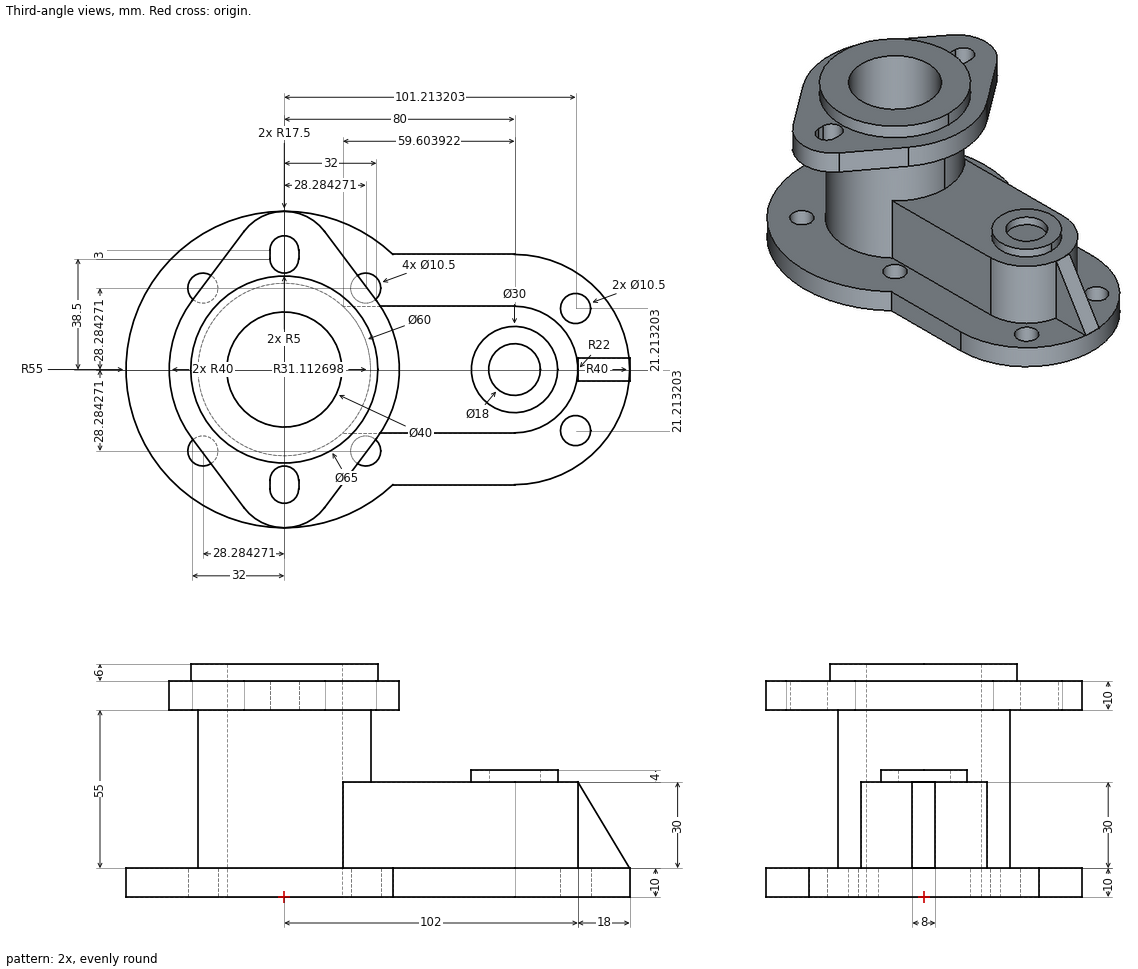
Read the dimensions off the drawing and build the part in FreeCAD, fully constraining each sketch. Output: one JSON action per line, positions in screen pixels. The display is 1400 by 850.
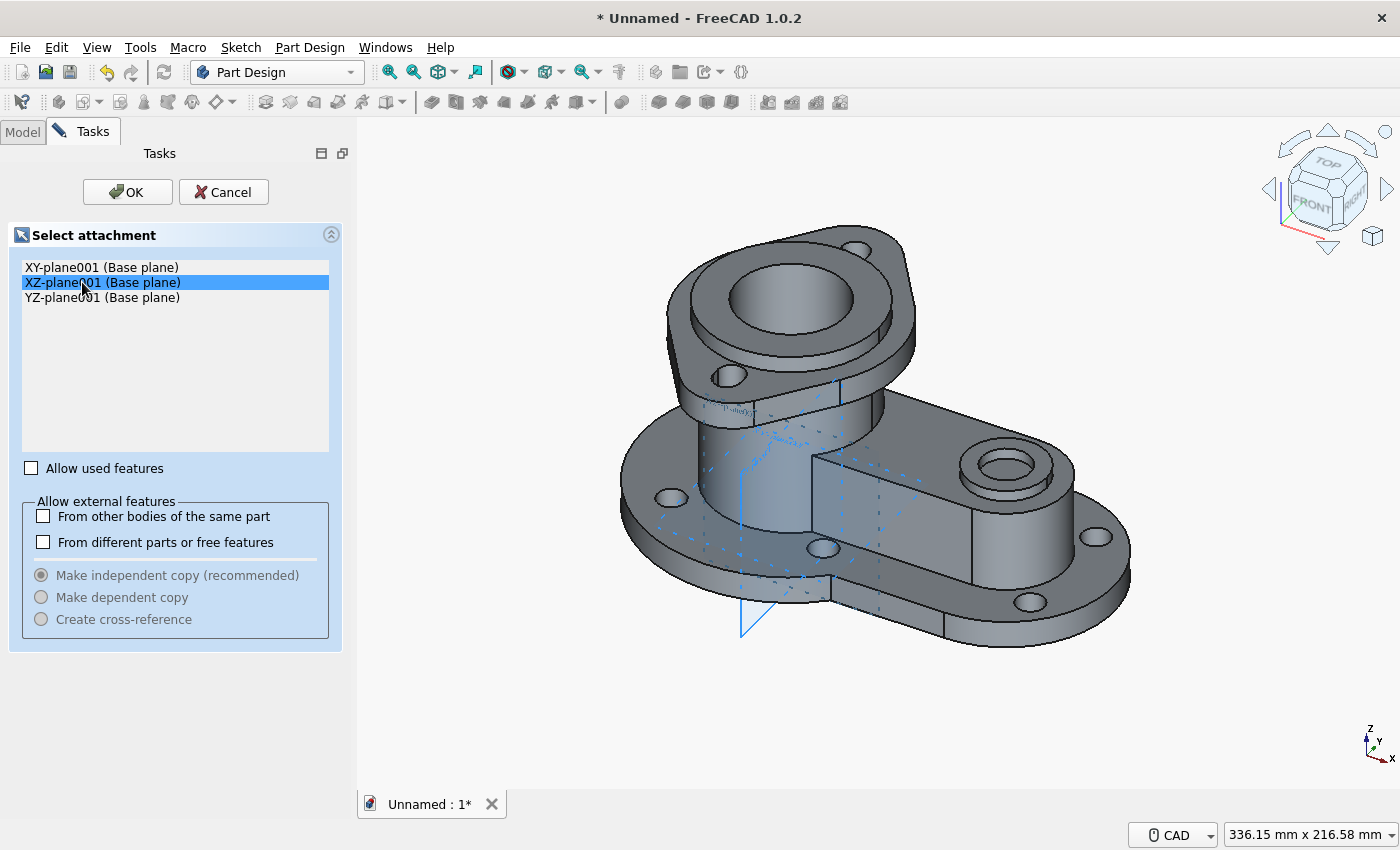
{"action": "left_click", "coordinate": [128, 192]}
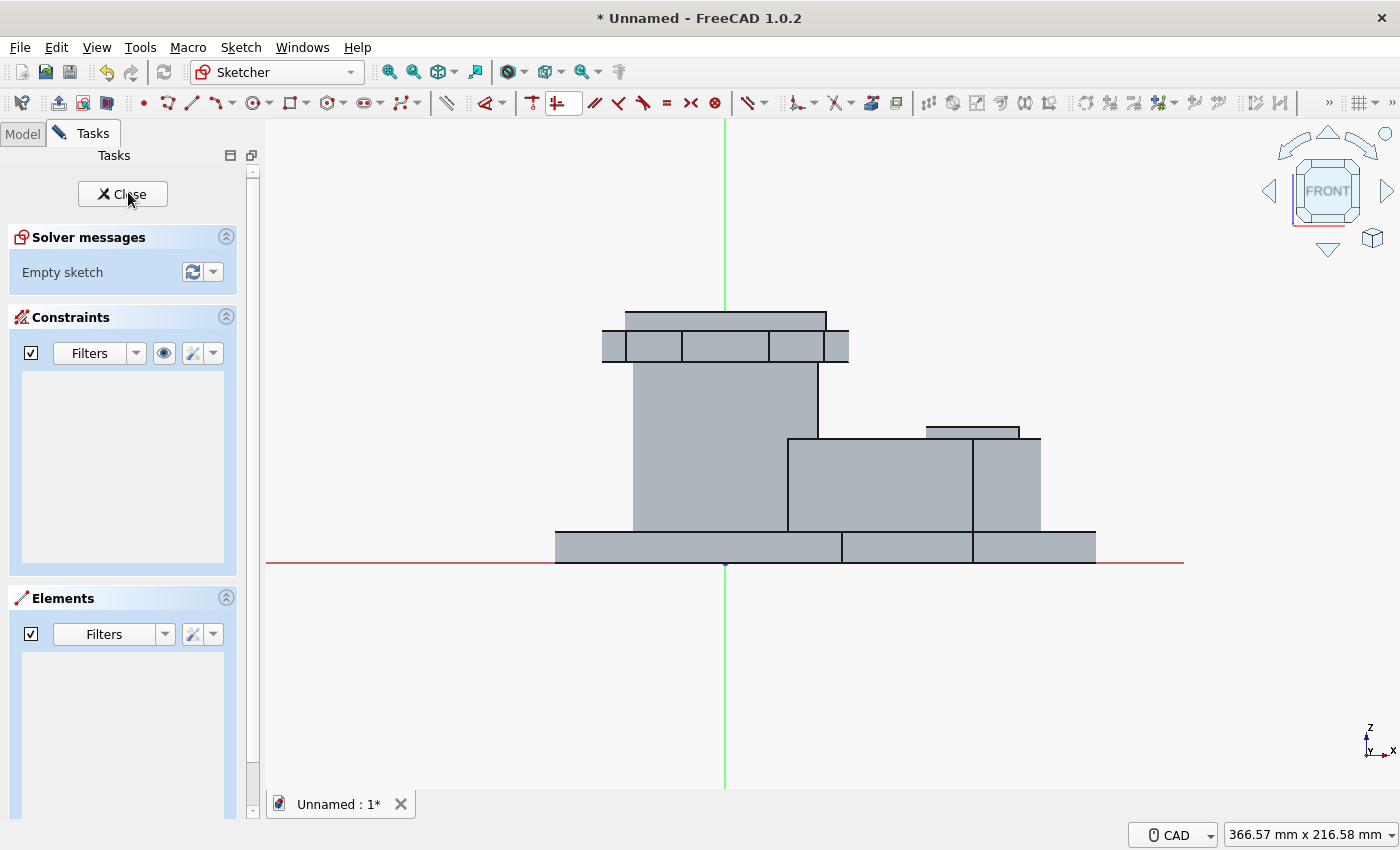
{"action": "scroll", "coordinate": [1146, 493], "scroll_direction": "up", "scroll_amount": 8}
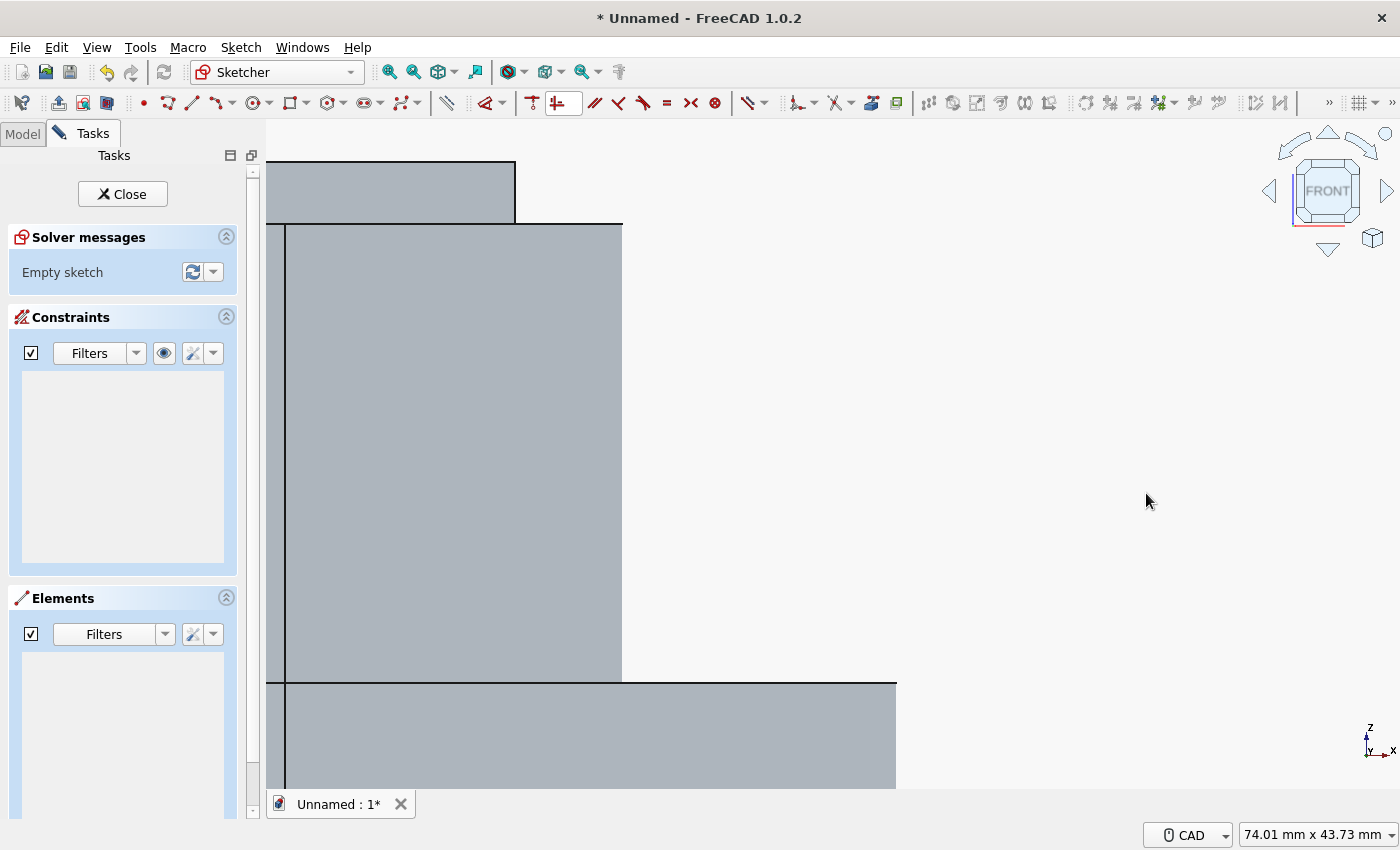
{"action": "left_click", "coordinate": [168, 104]}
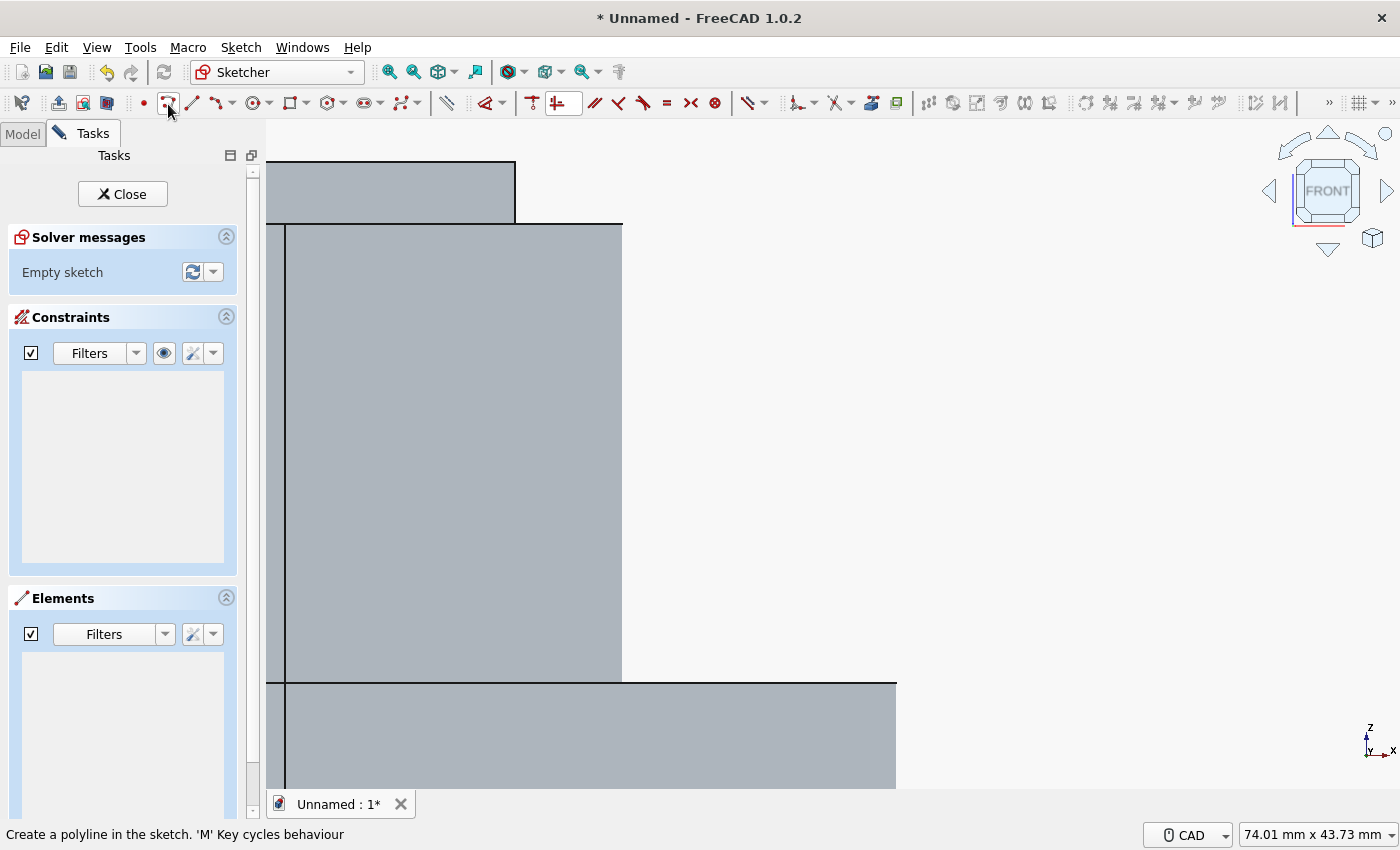
{"action": "left_click", "coordinate": [622, 683]}
{"action": "left_click", "coordinate": [622, 224]}
{"action": "left_click", "coordinate": [898, 683]}
{"action": "left_click", "coordinate": [622, 684]}
{"action": "key", "text": "Escape"}
{"action": "key", "text": "Escape"}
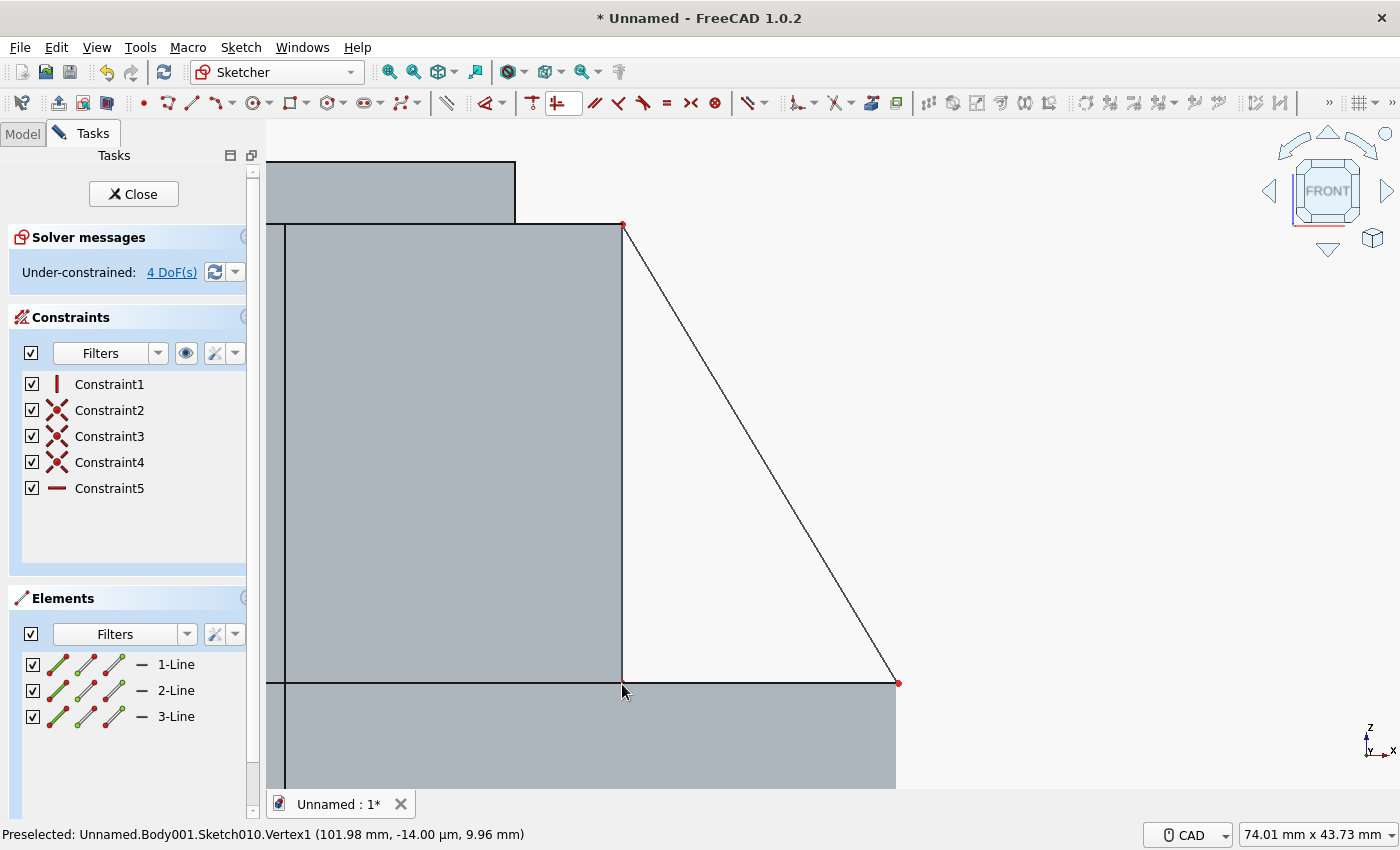
{"action": "key", "text": "d"}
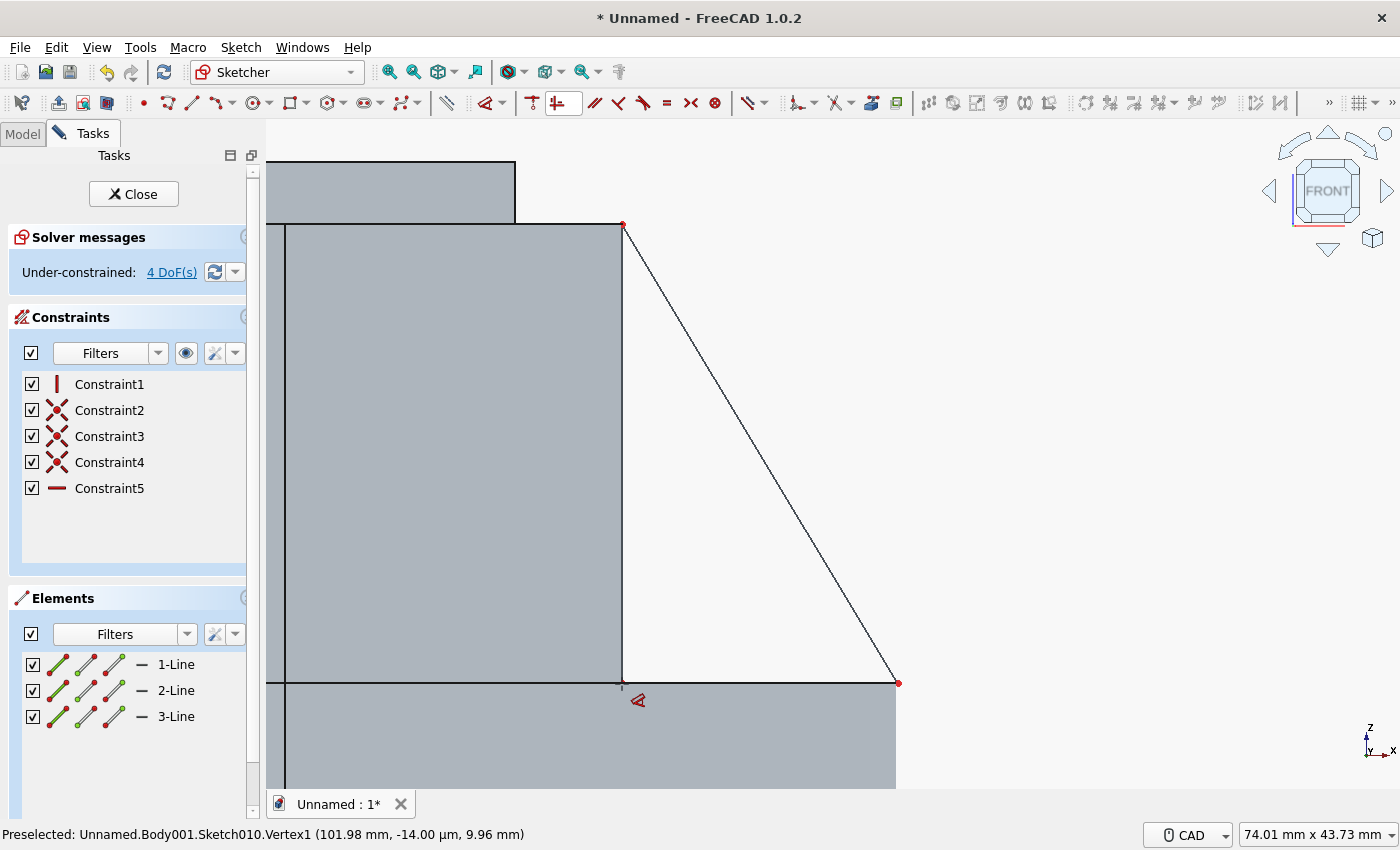
{"action": "left_click", "coordinate": [622, 546]}
{"action": "left_click", "coordinate": [588, 454]}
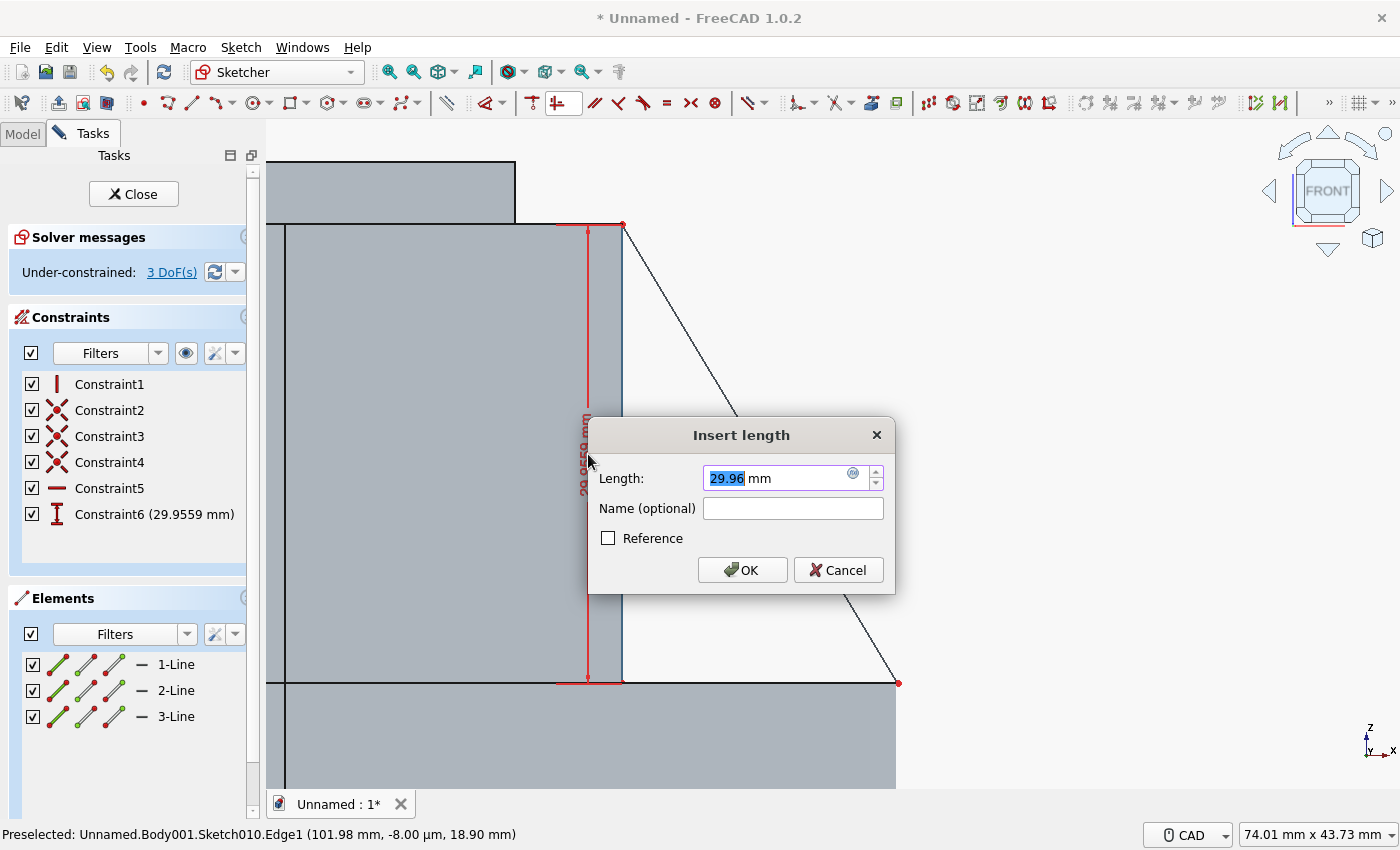
{"action": "type", "text": "30"}
{"action": "key", "text": "Return"}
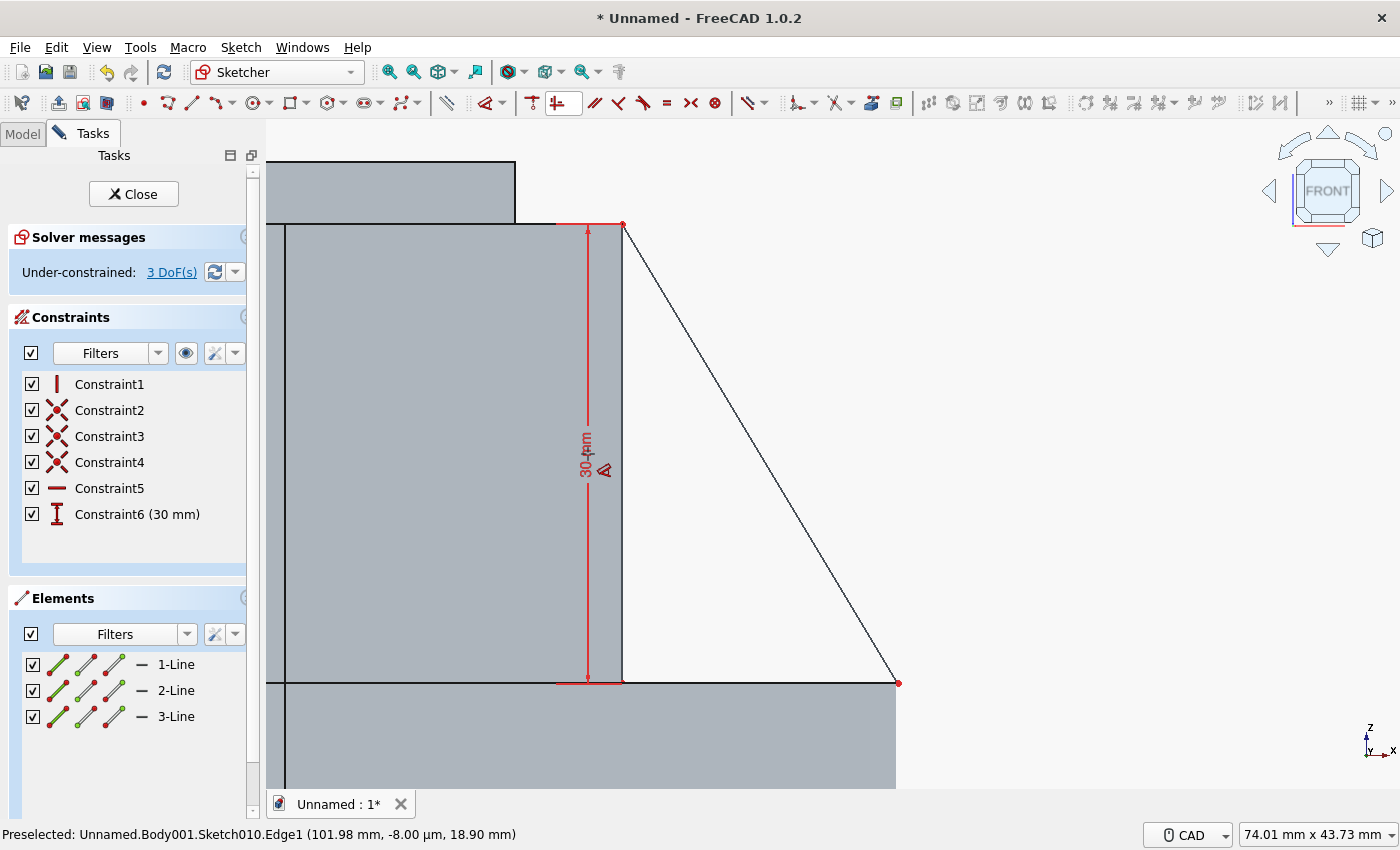
{"action": "left_click", "coordinate": [815, 684]}
{"action": "left_click", "coordinate": [760, 718]}